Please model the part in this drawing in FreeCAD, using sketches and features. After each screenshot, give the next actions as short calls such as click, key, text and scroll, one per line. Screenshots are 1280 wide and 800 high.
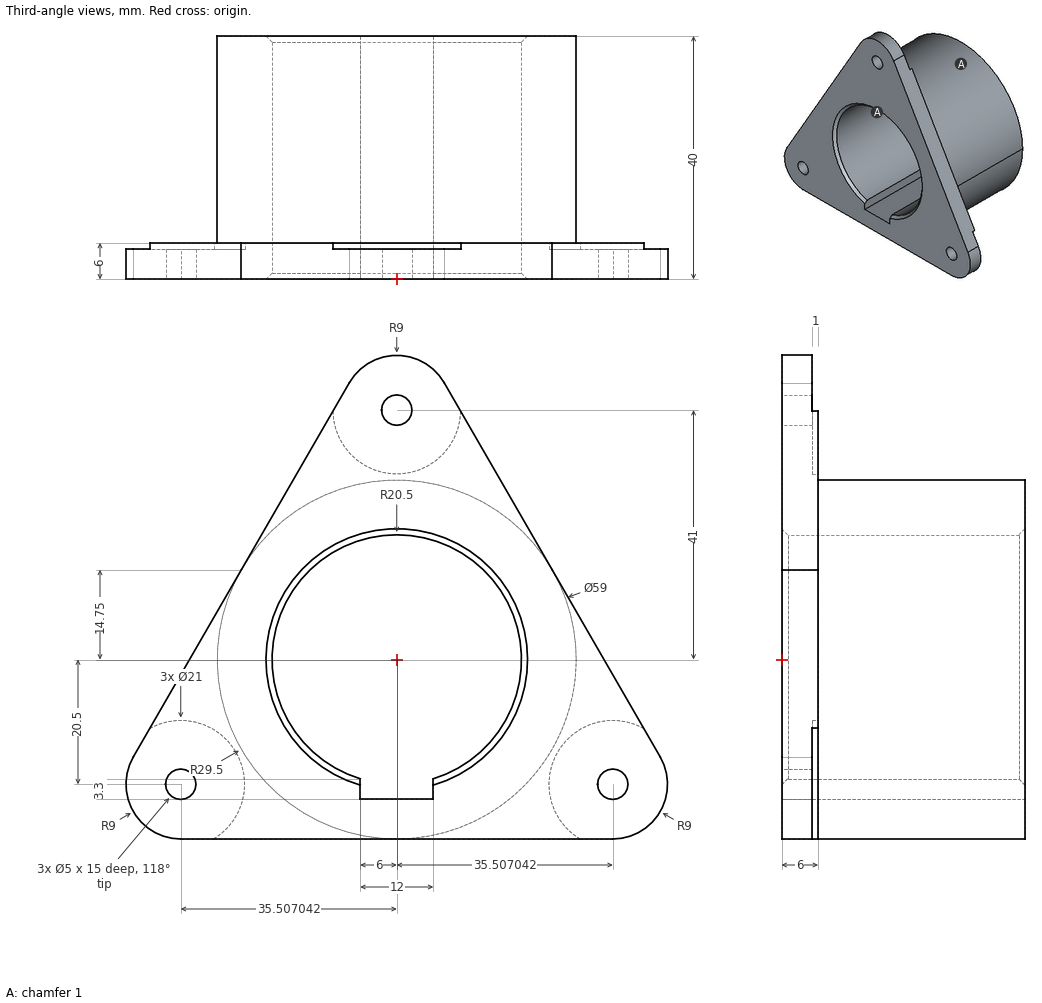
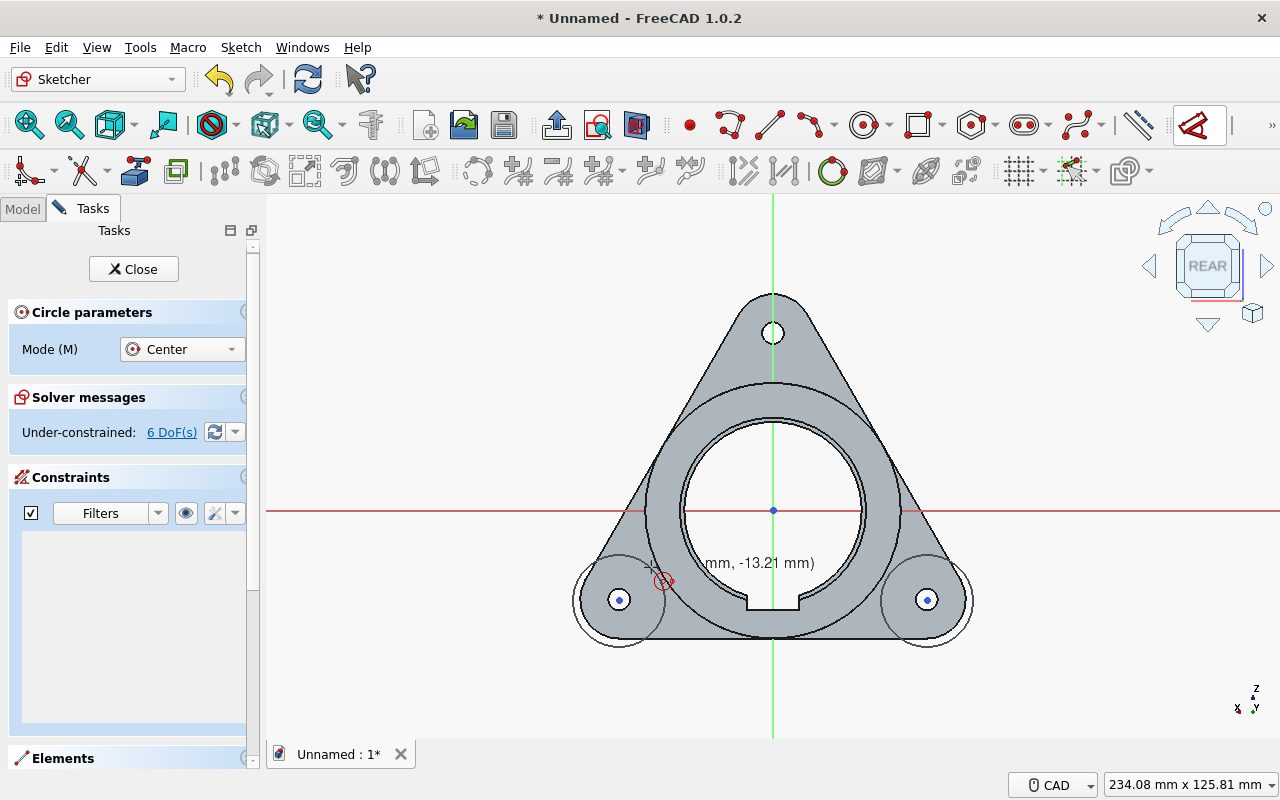
click(773, 333)
click(805, 301)
key(Escape)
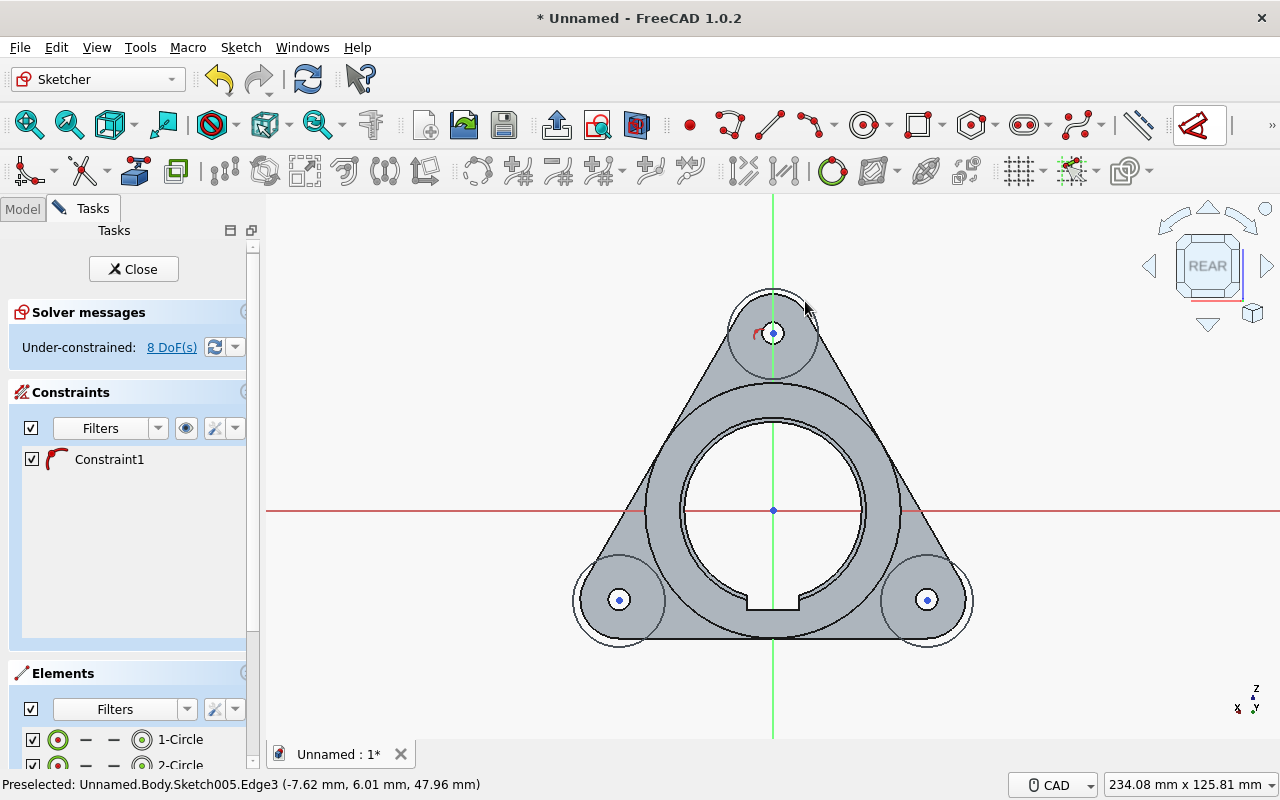
click(959, 568)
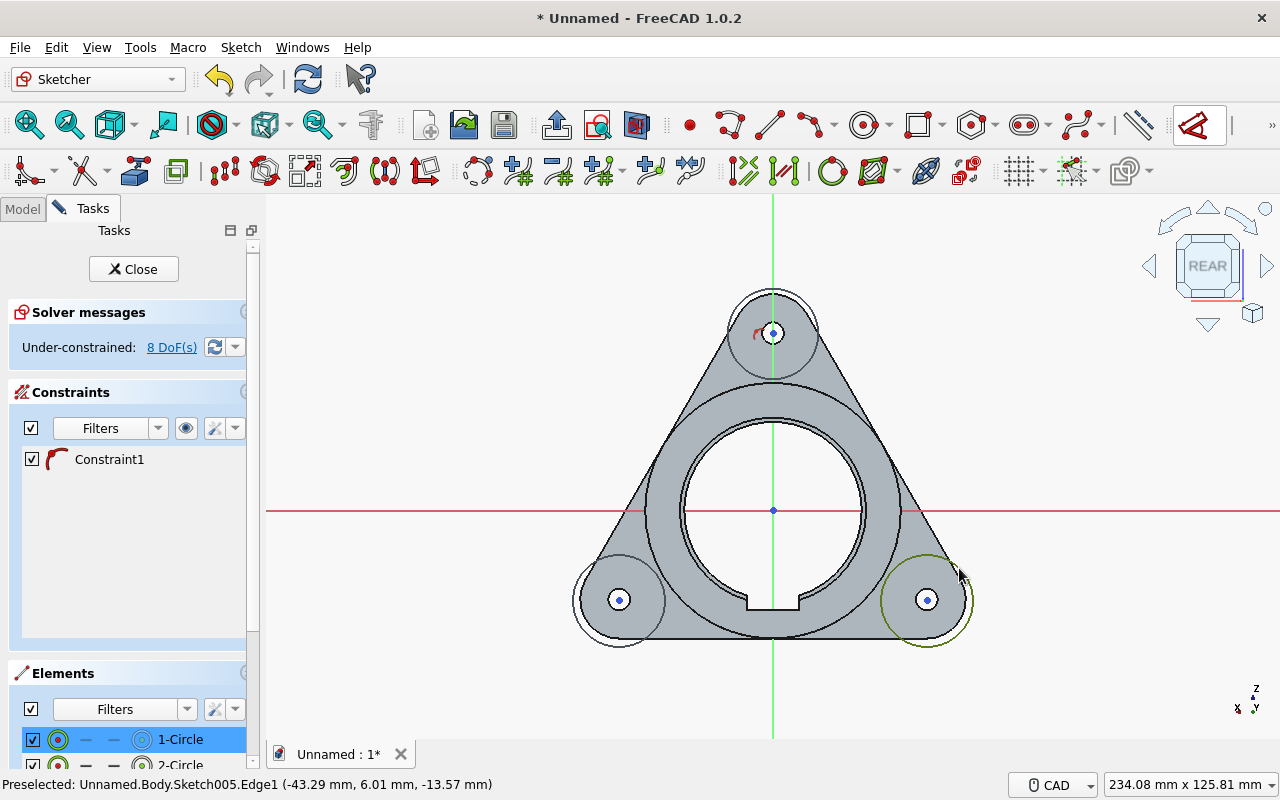
click(651, 568)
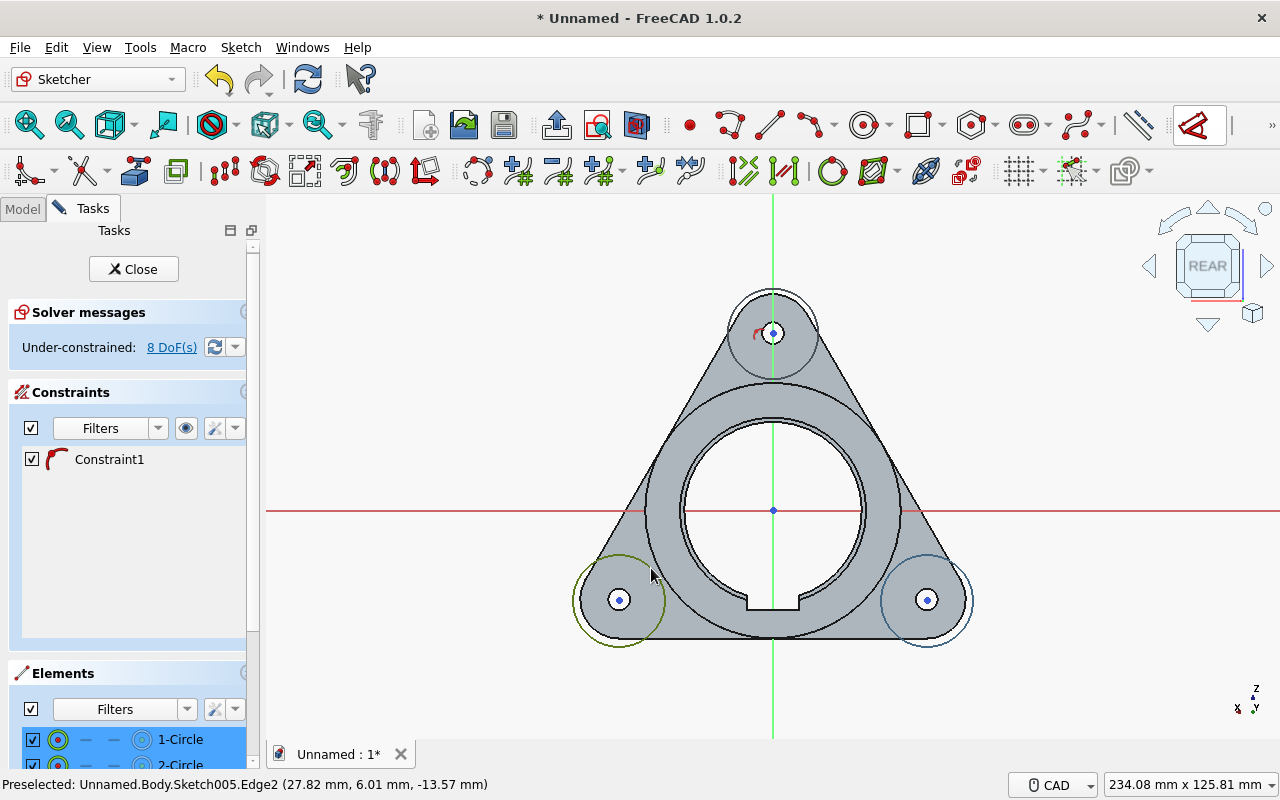
click(805, 302)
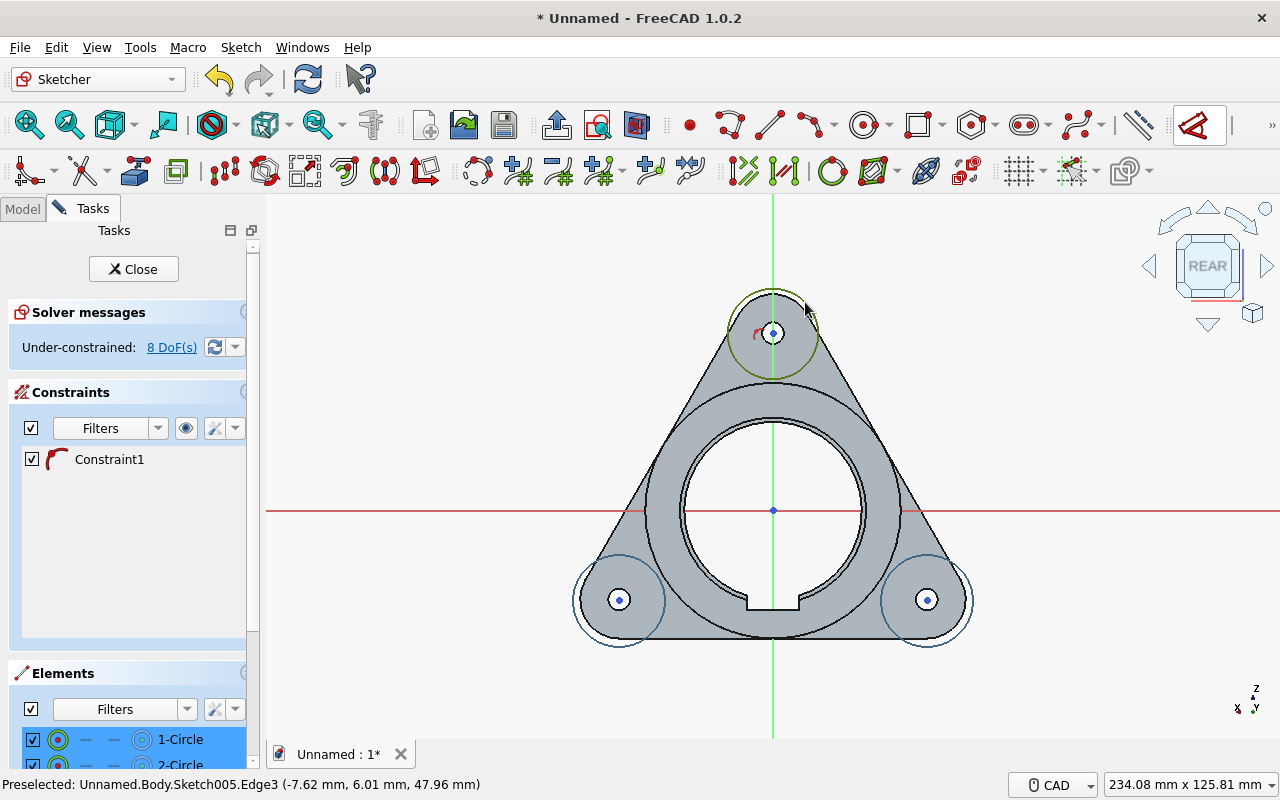
key(e)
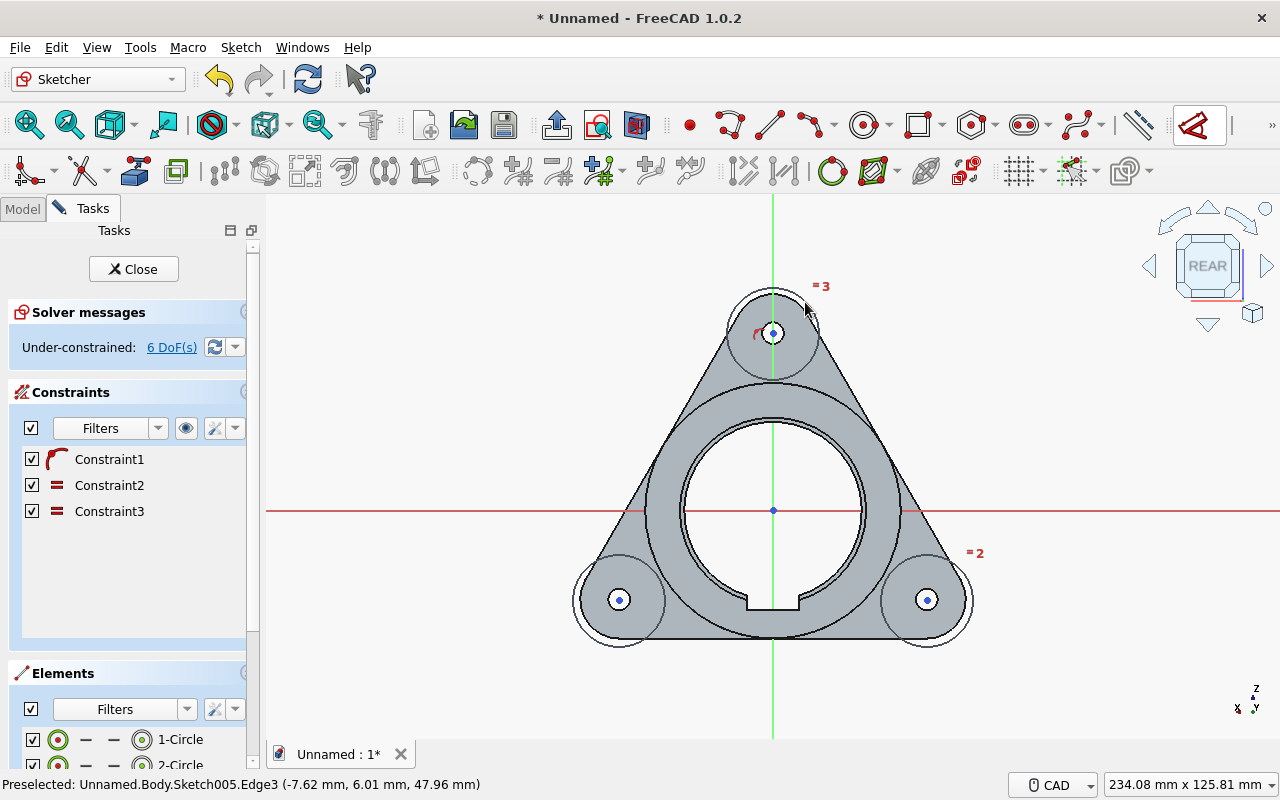
click(927, 601)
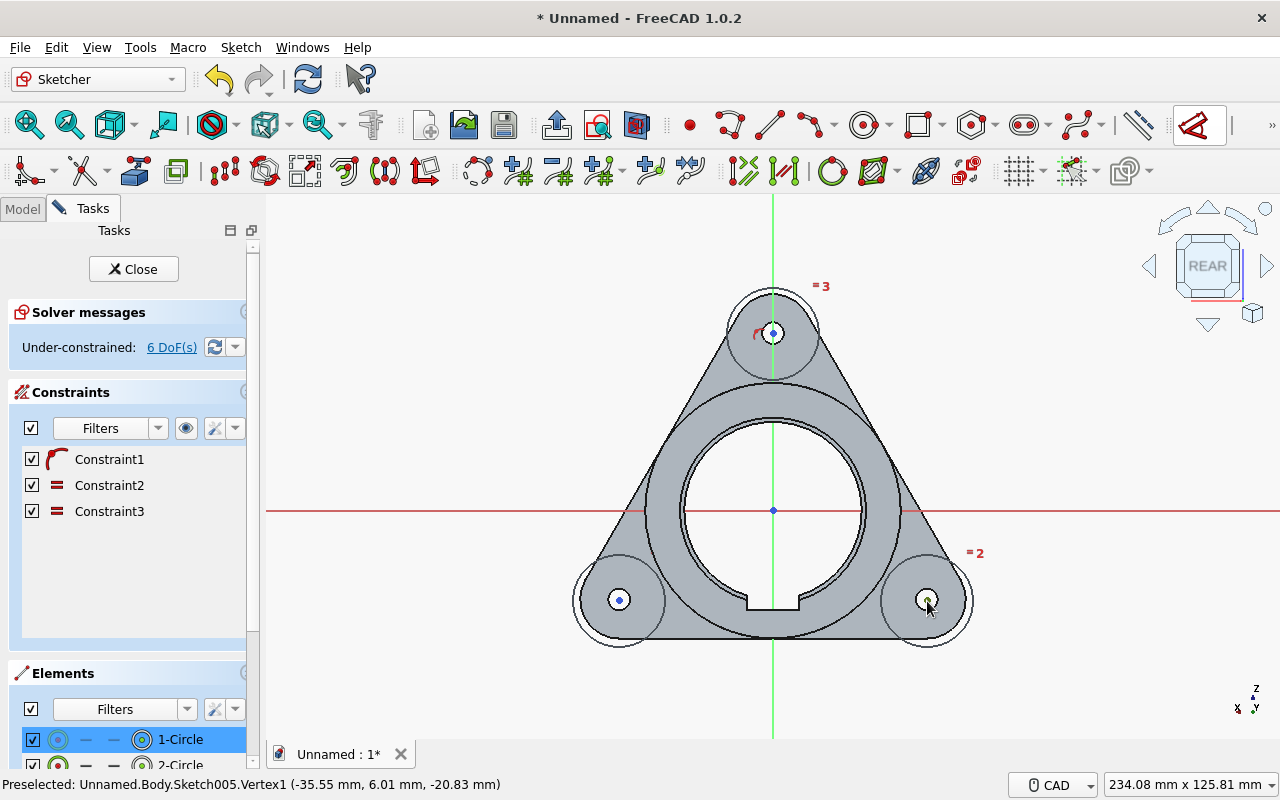
click(619, 601)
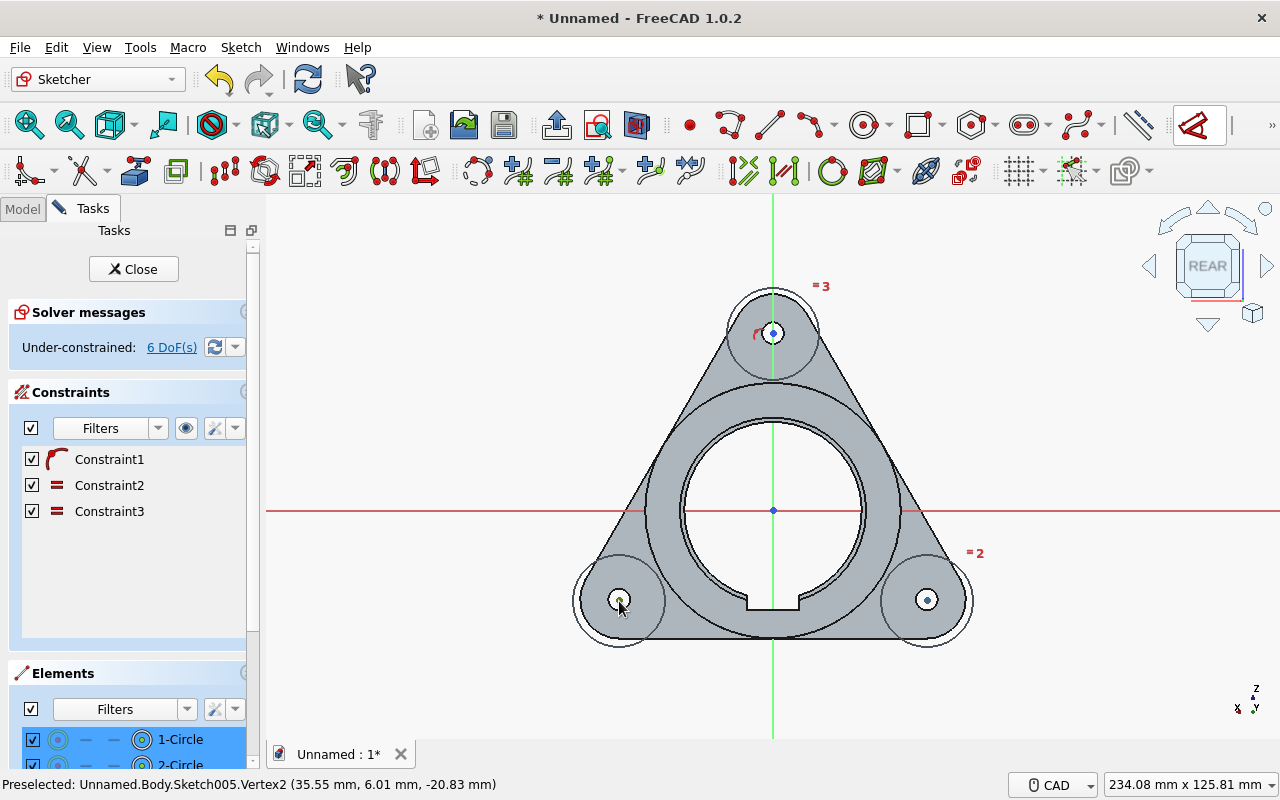
key(h)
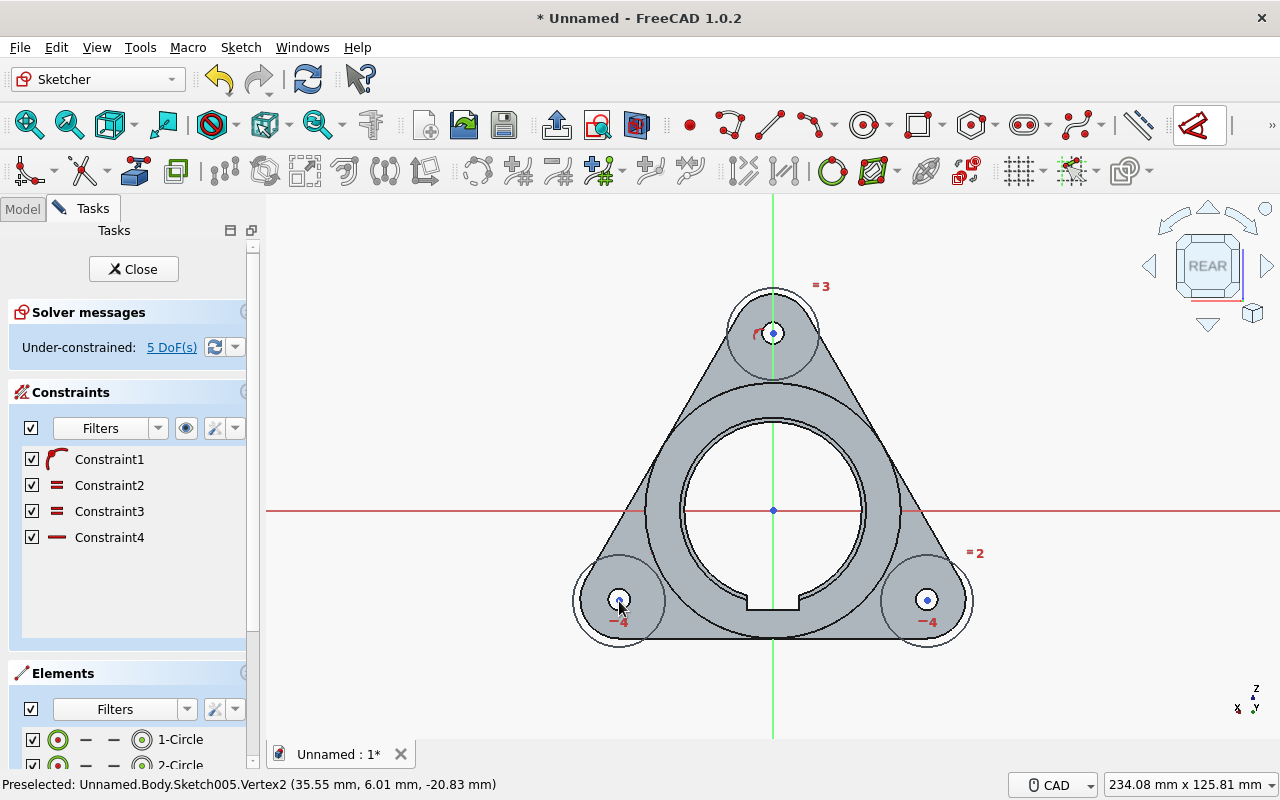
click(959, 568)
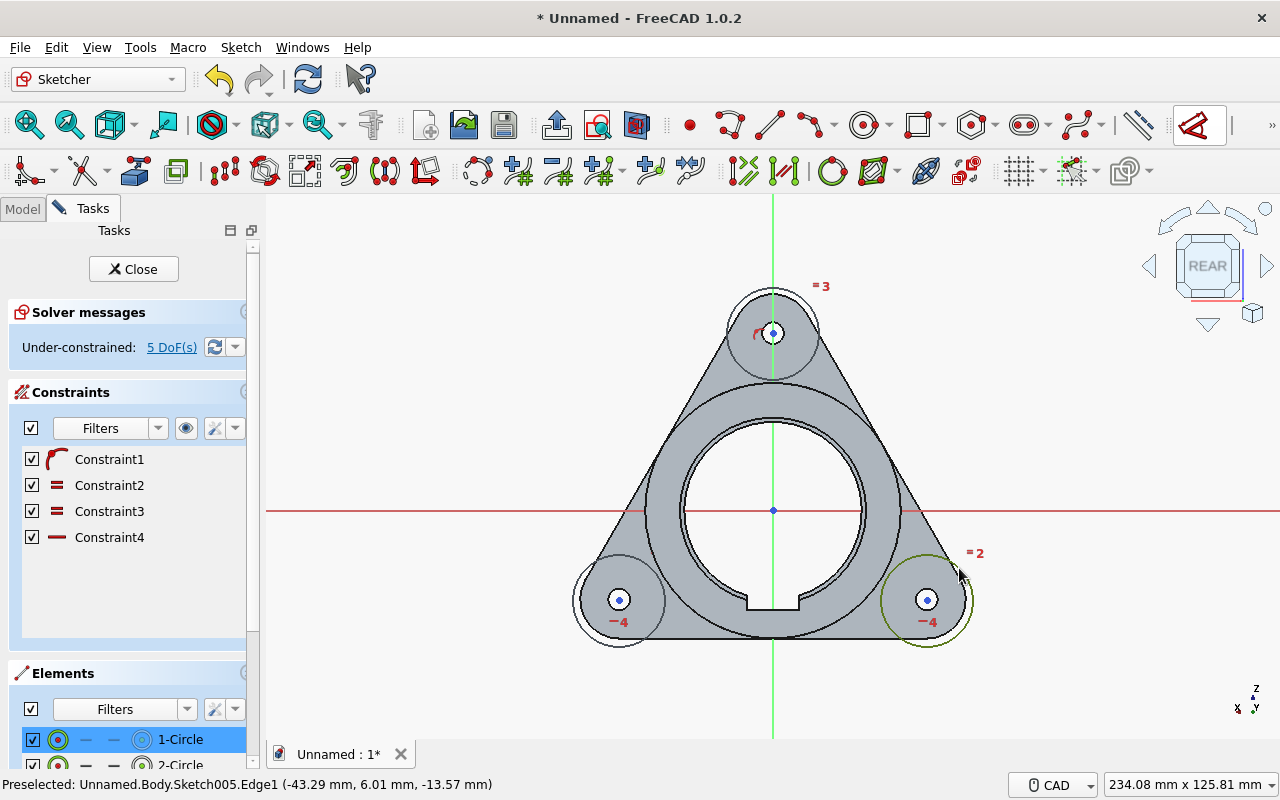
click(1220, 126)